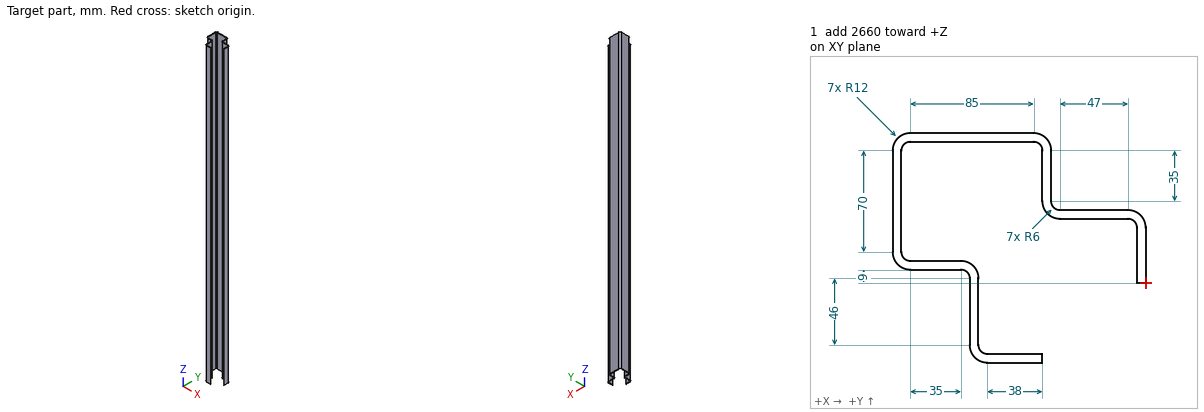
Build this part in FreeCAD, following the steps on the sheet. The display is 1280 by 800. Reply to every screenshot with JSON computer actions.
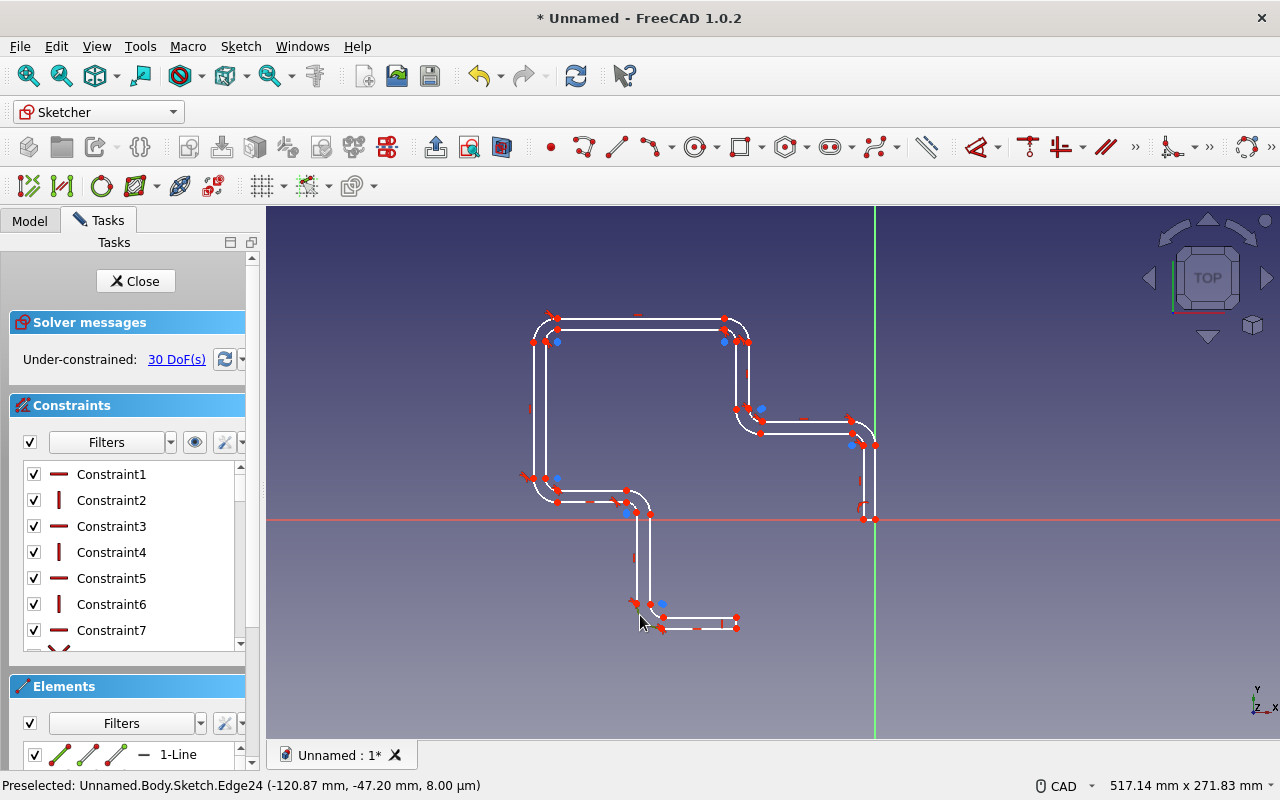
{"action": "scroll", "coordinate": [654, 614], "scroll_direction": "up", "scroll_amount": 2}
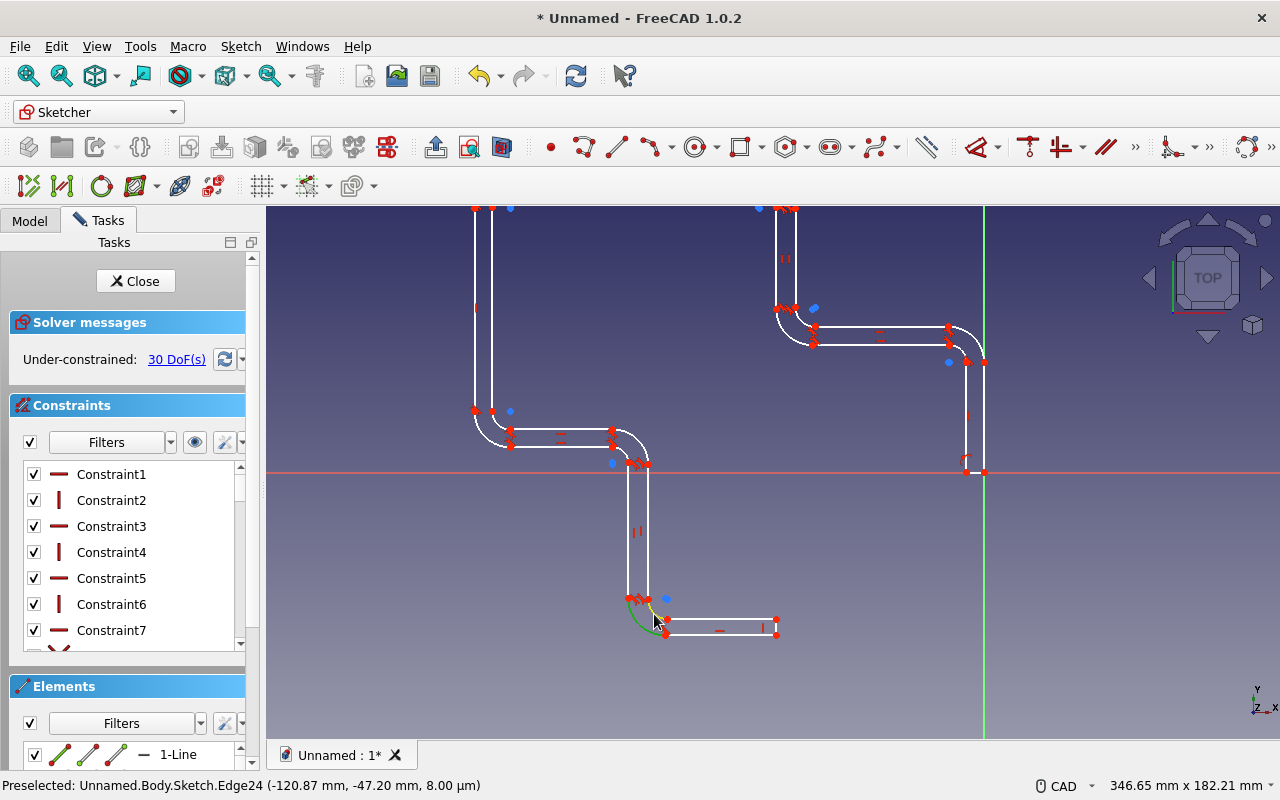
{"action": "left_click", "coordinate": [654, 613]}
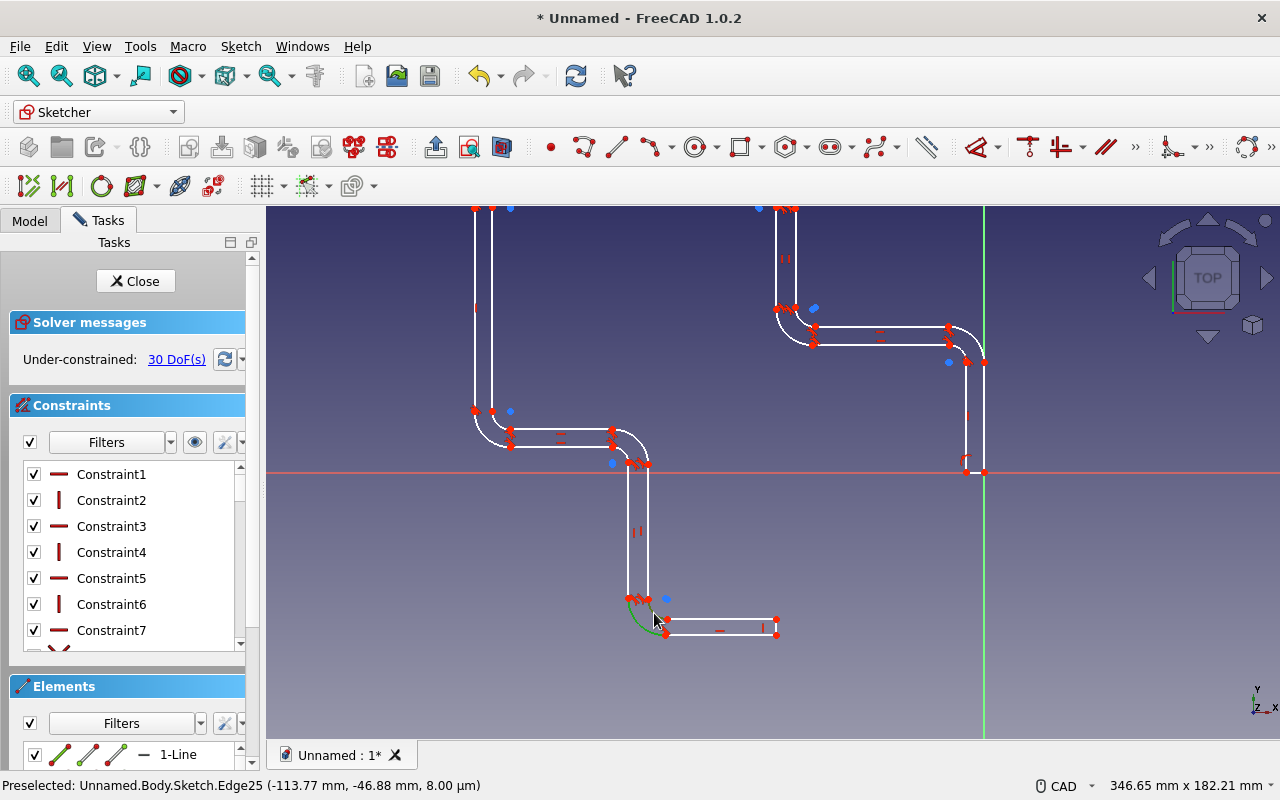
{"action": "key", "text": "c"}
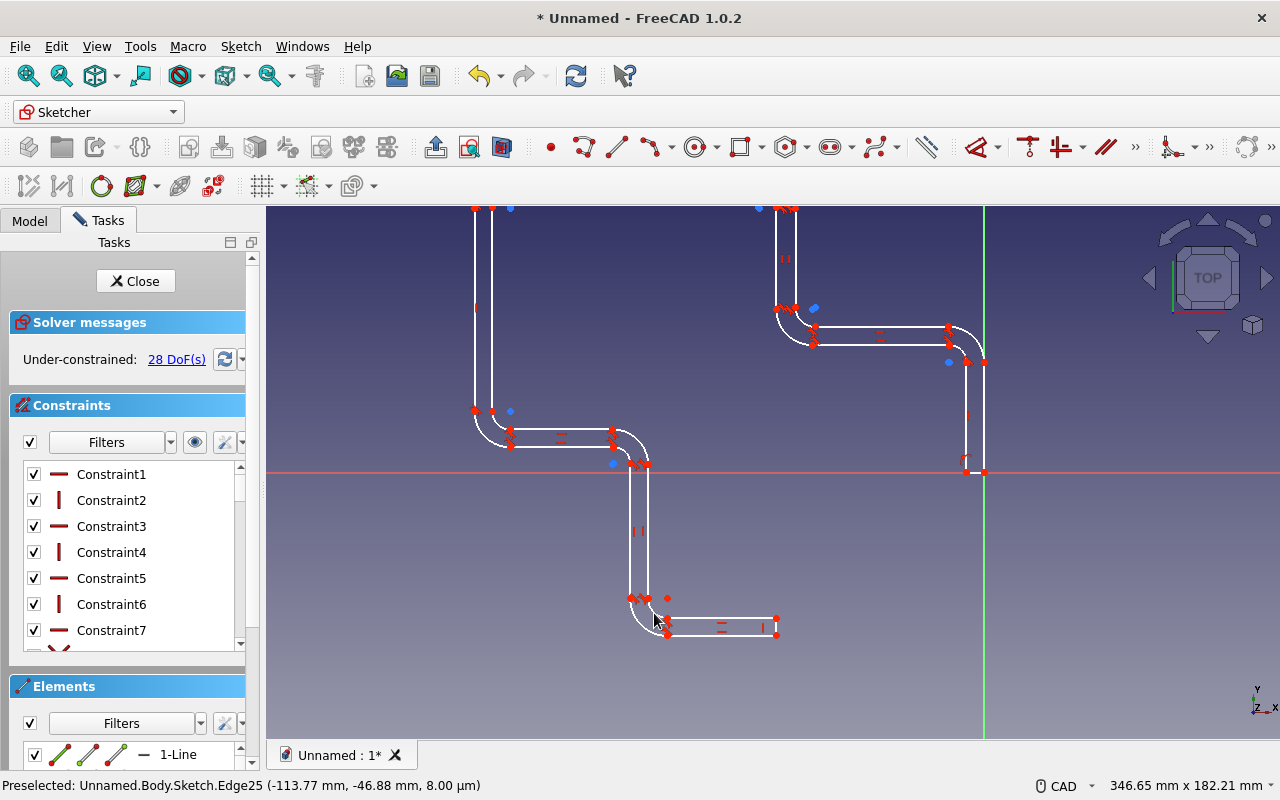
{"action": "left_click", "coordinate": [625, 452]}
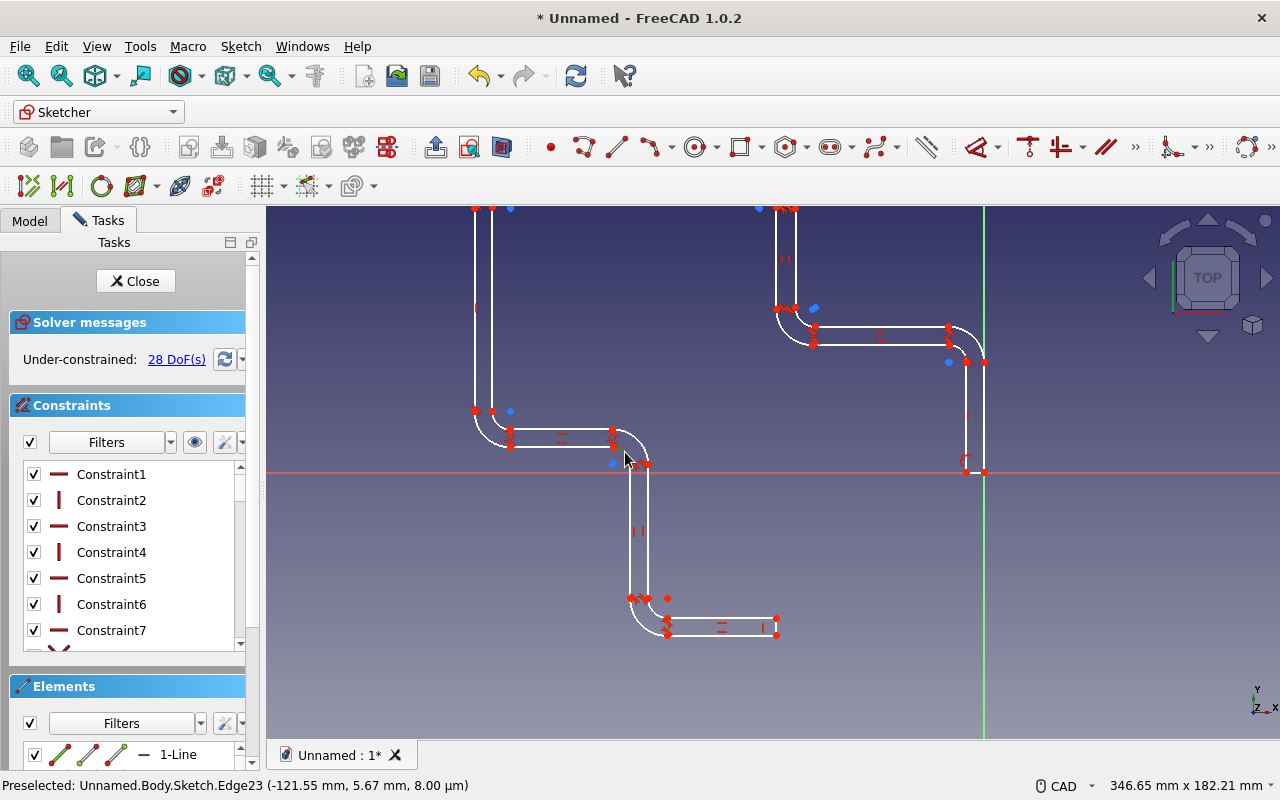
{"action": "left_click", "coordinate": [644, 449]}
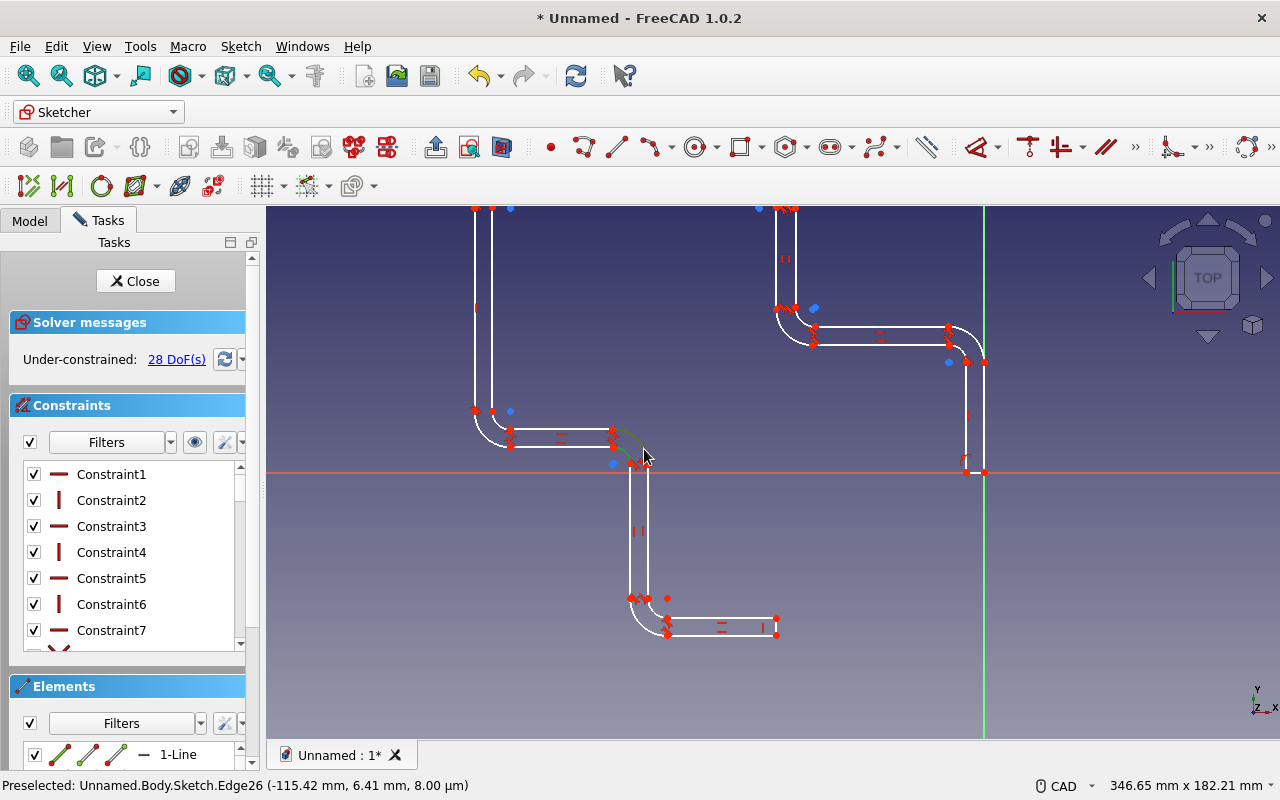
{"action": "key", "text": "c"}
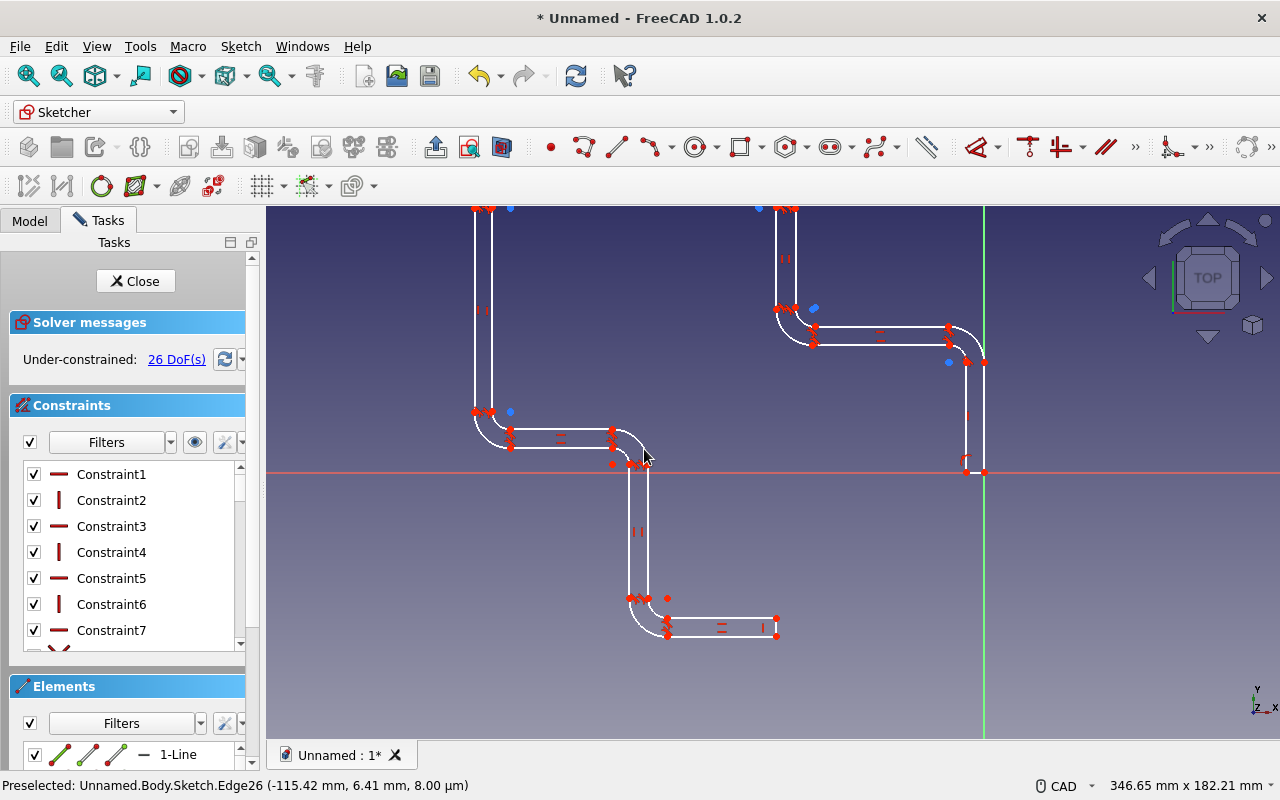
{"action": "left_click", "coordinate": [478, 429]}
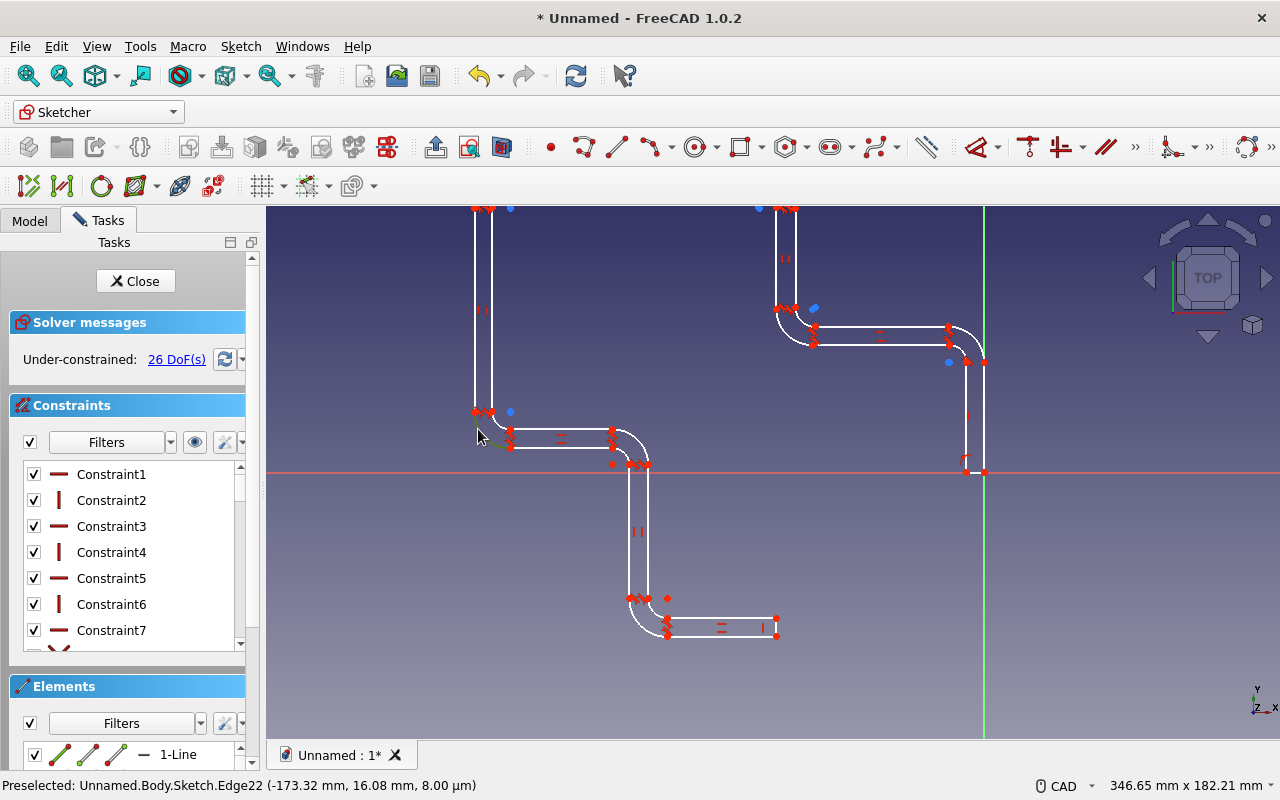
{"action": "left_click", "coordinate": [498, 424]}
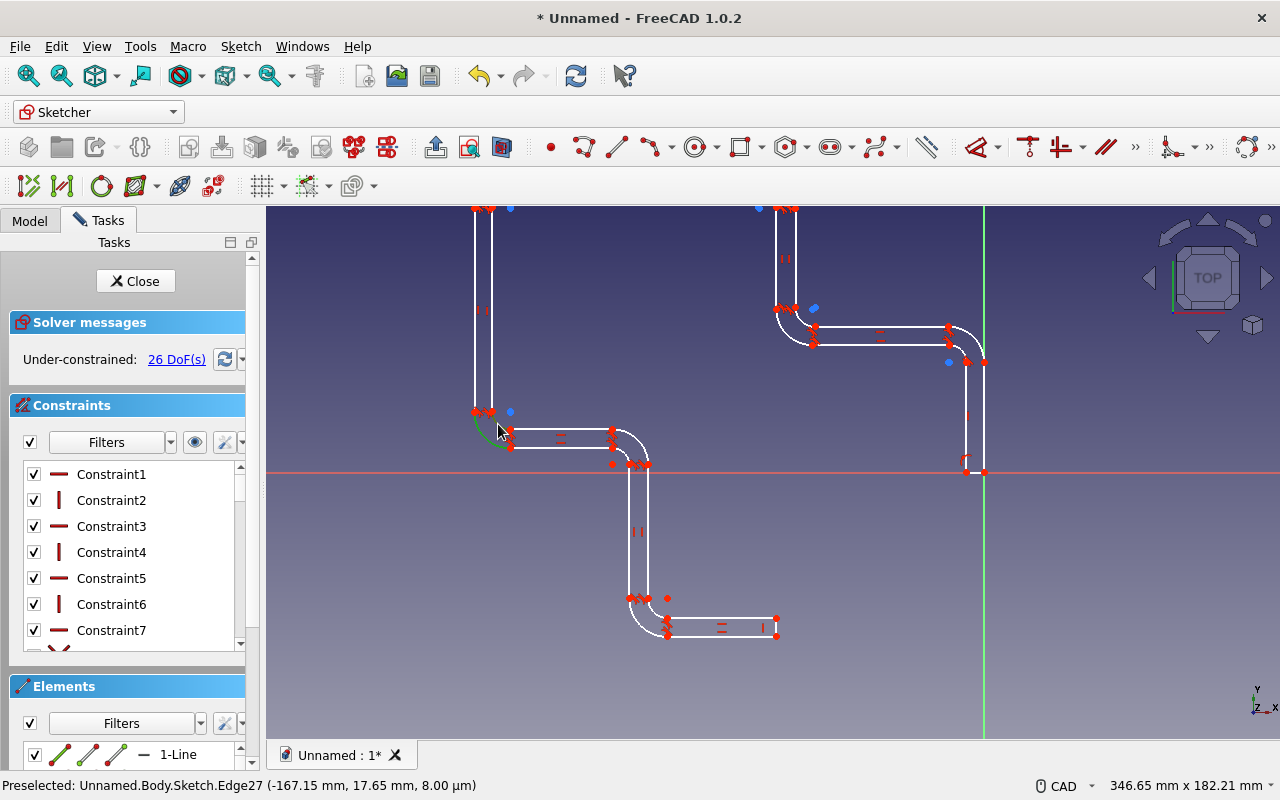
{"action": "key", "text": "c"}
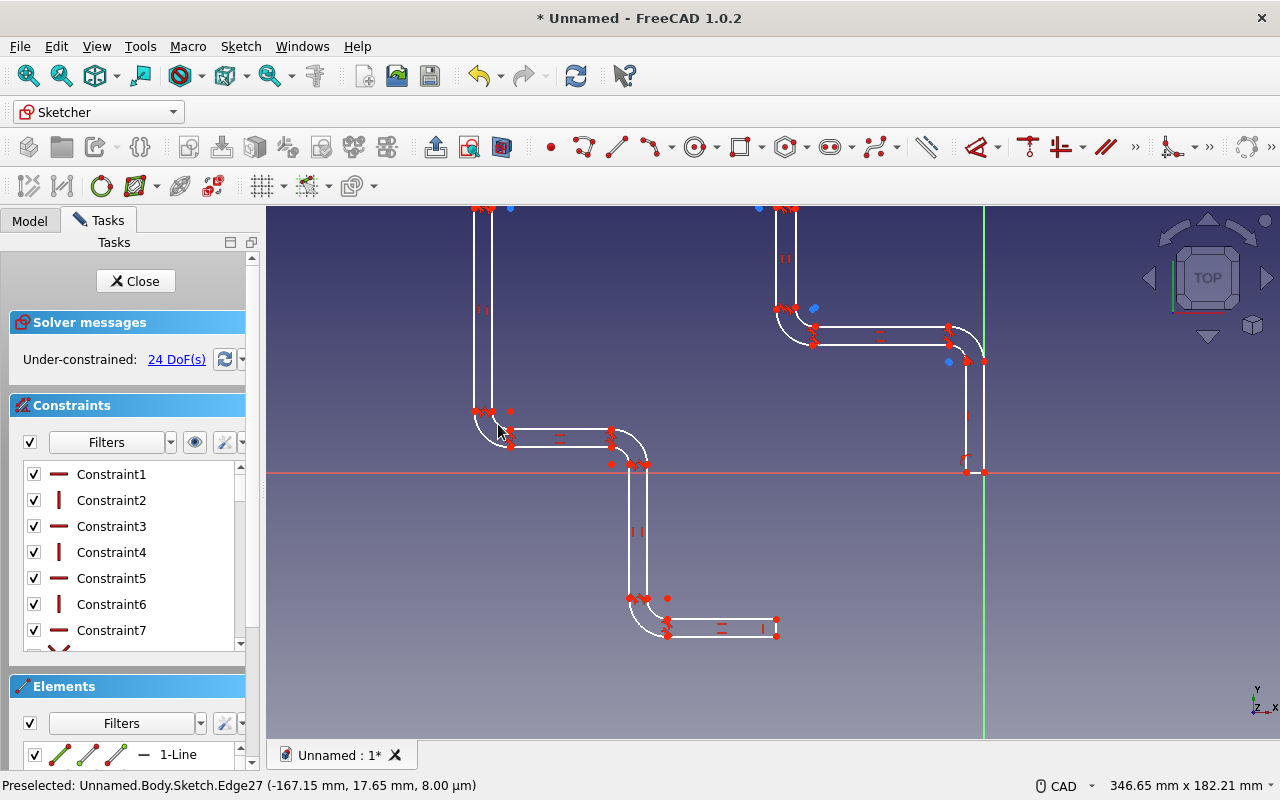
{"action": "scroll", "coordinate": [654, 615], "scroll_direction": "down", "scroll_amount": 2}